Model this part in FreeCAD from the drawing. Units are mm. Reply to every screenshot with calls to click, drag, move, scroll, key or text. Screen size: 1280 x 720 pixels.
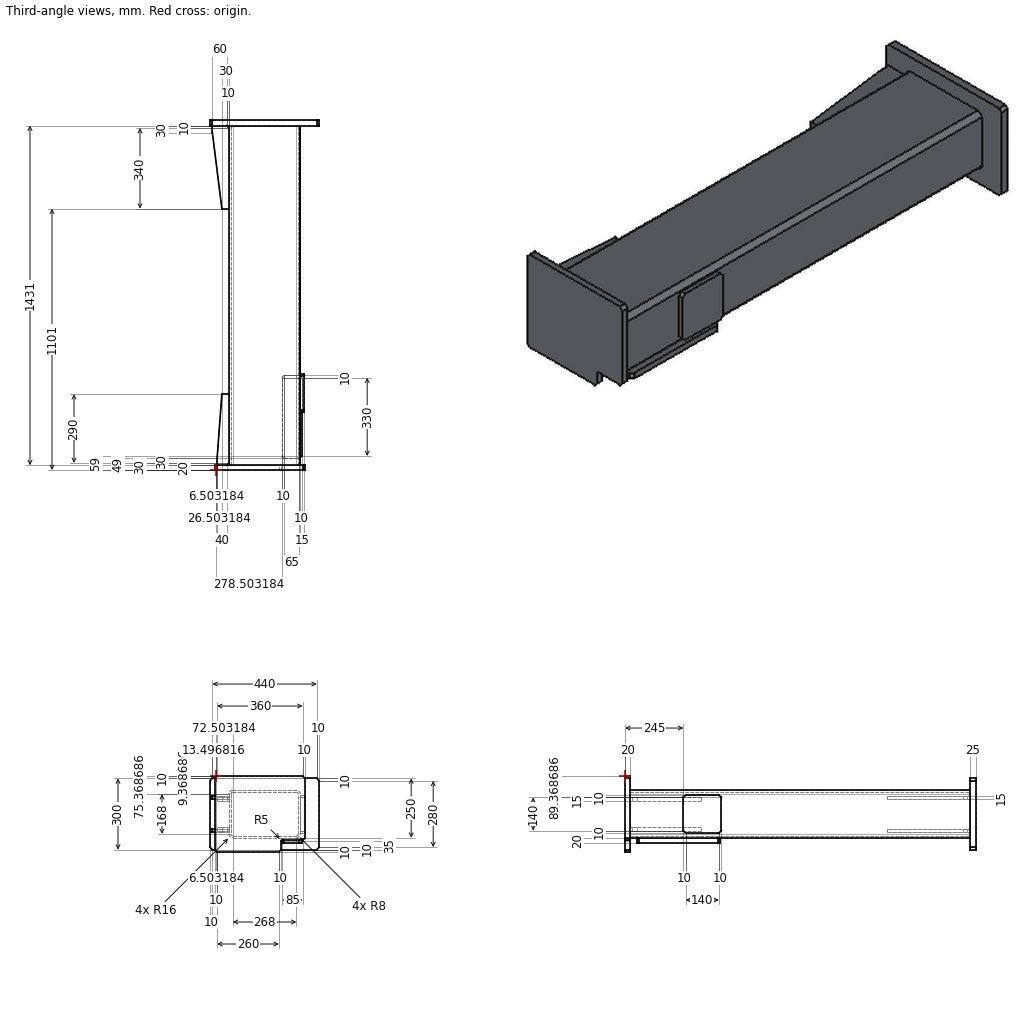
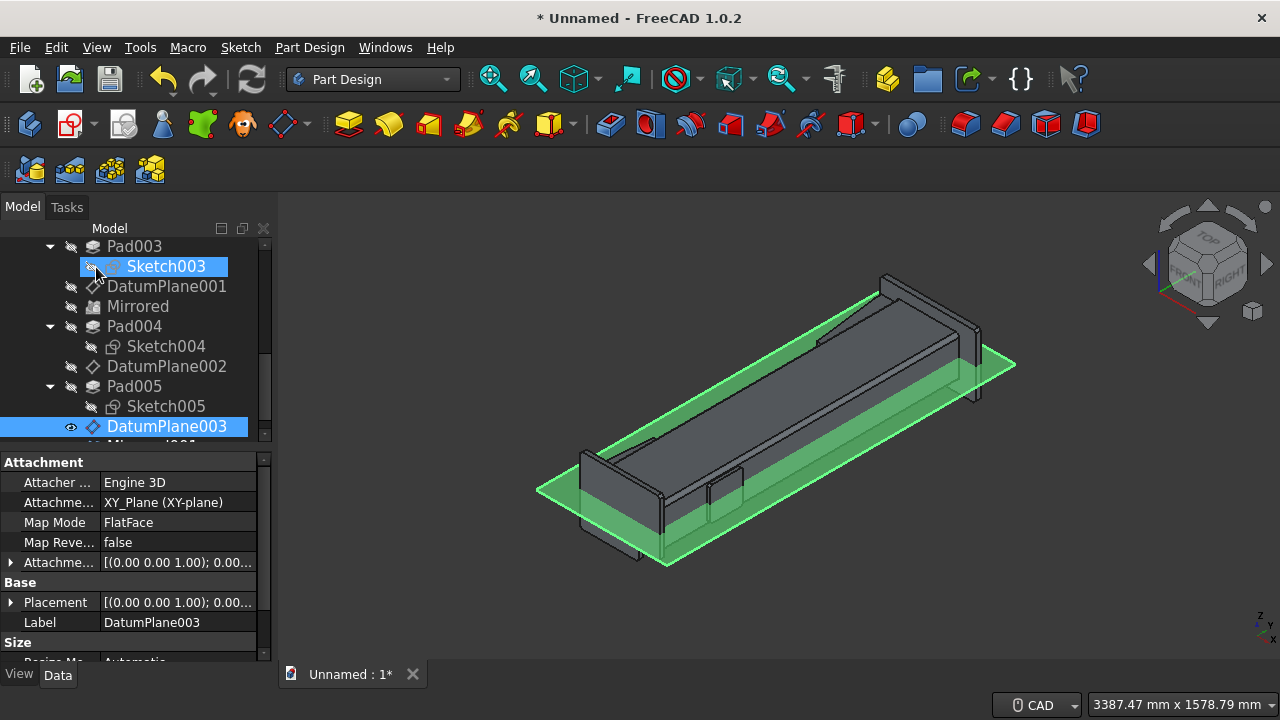
click(116, 427)
key(space)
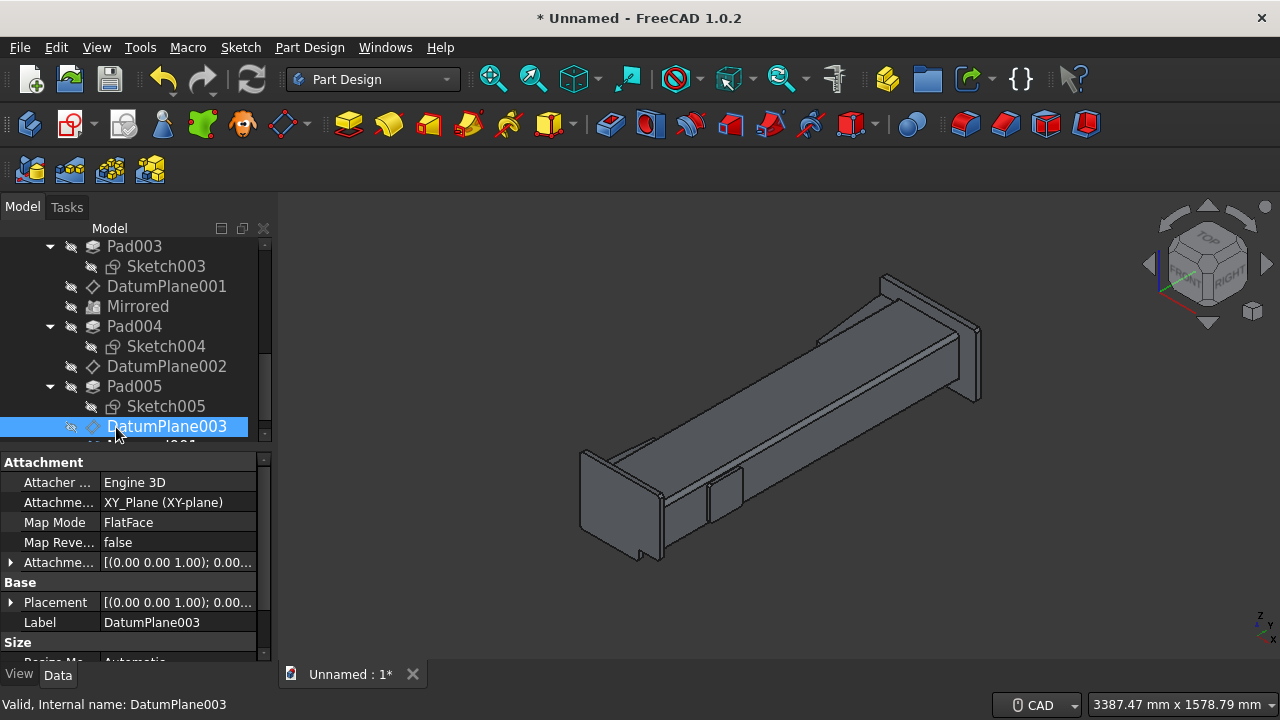
key(5)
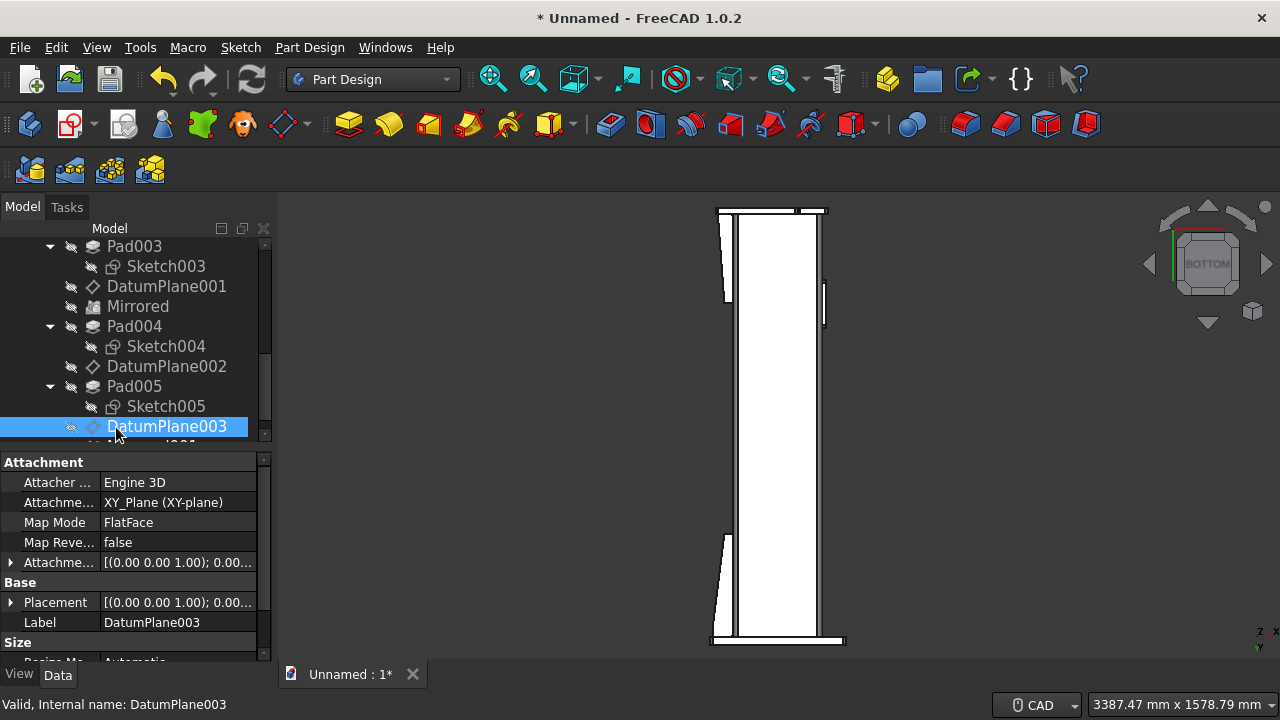
click(778, 545)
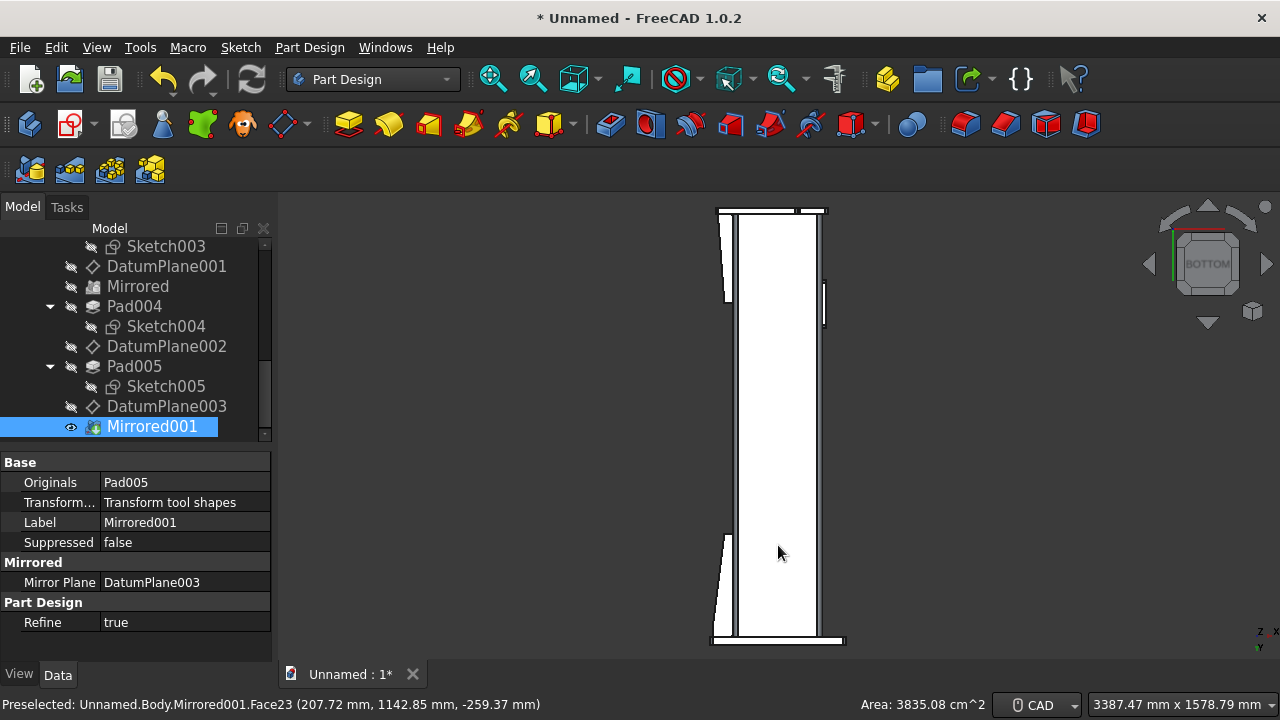
click(70, 124)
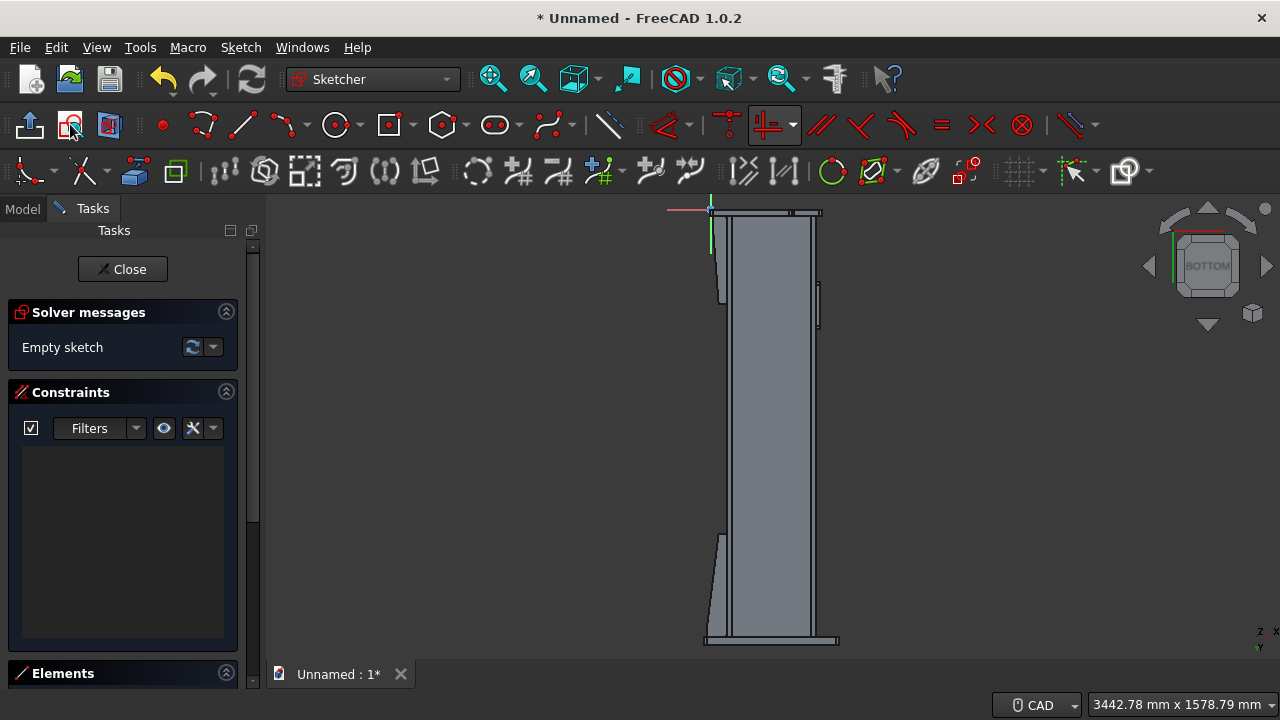
key(q)
key(s)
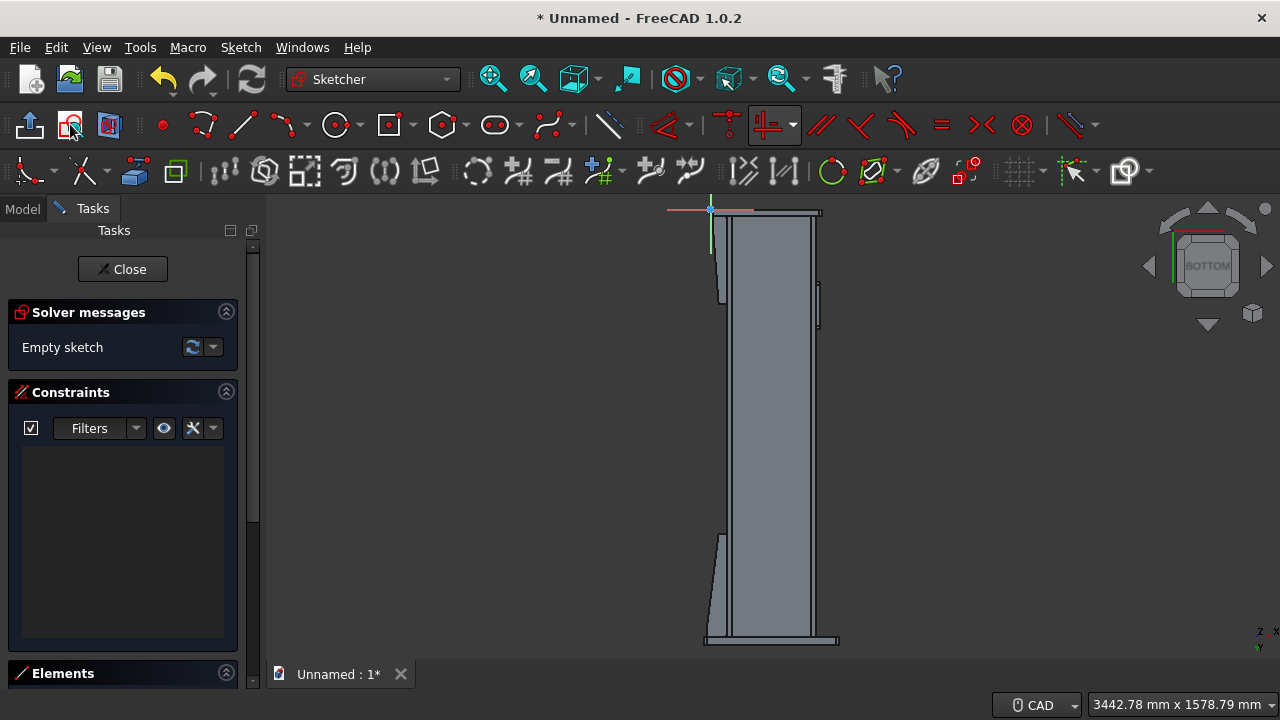
scroll(704, 426, down, 5)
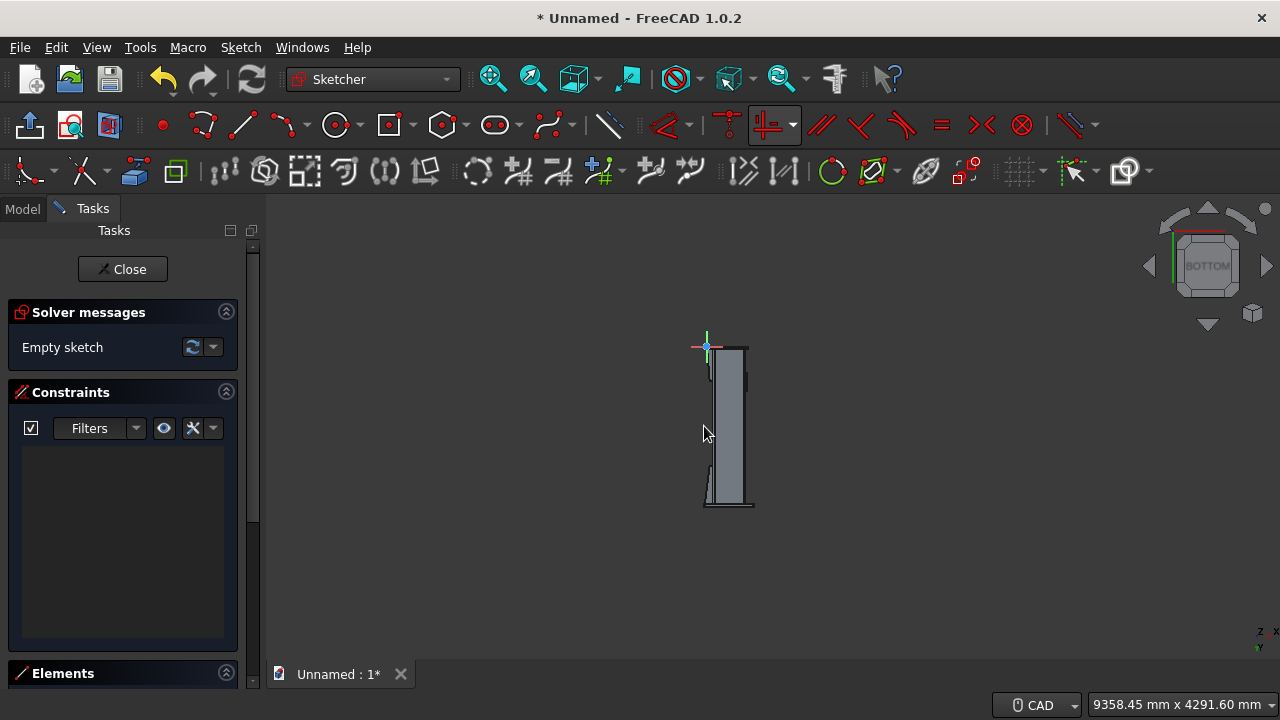
scroll(731, 357, up, 9)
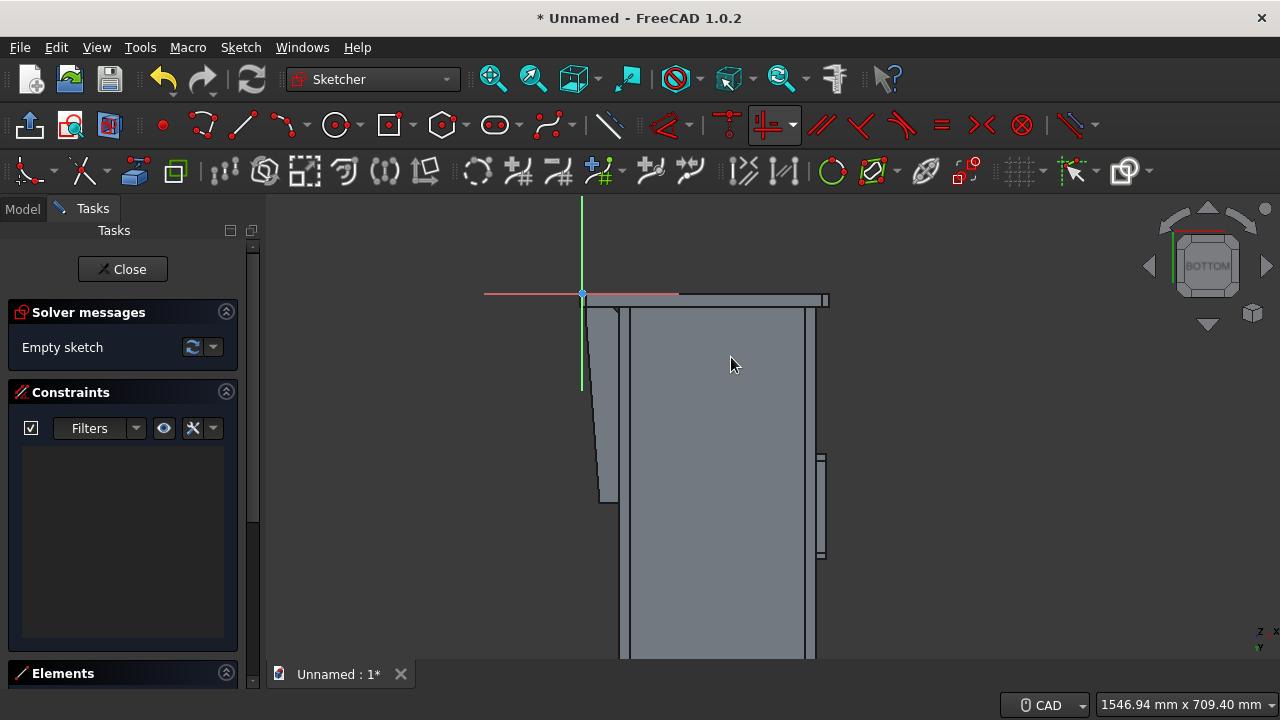
click(204, 126)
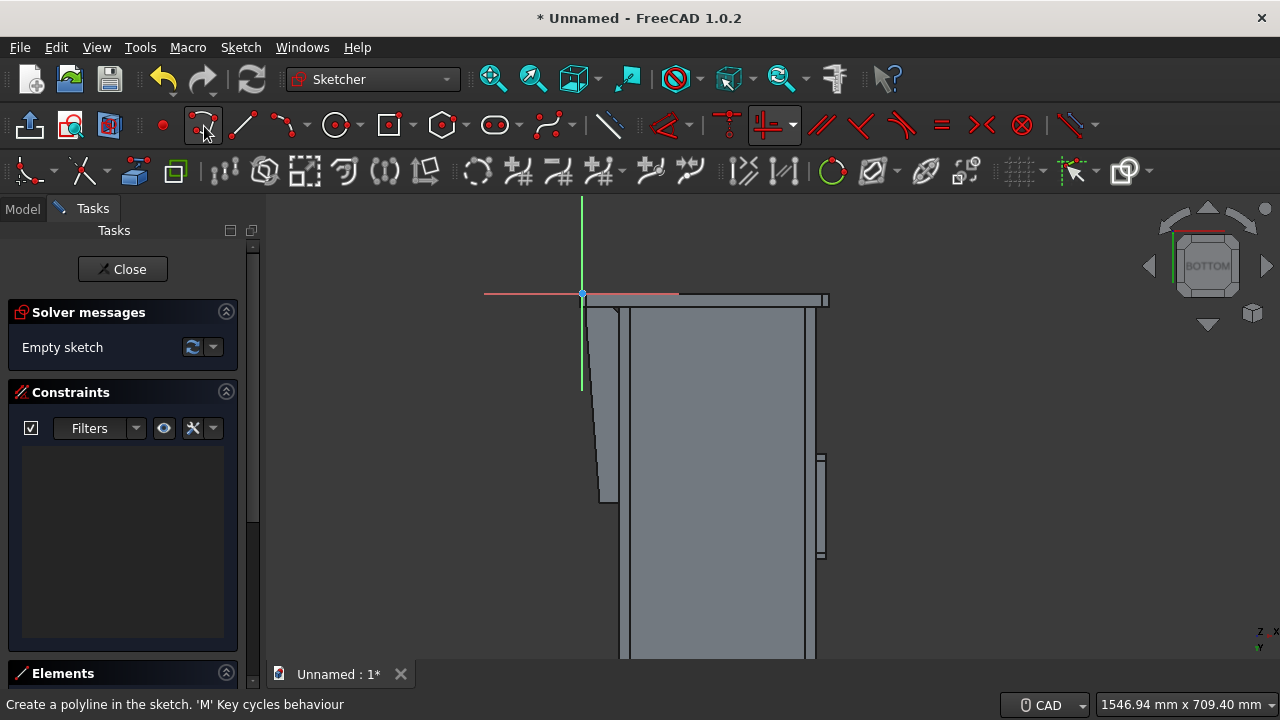
click(765, 332)
click(765, 549)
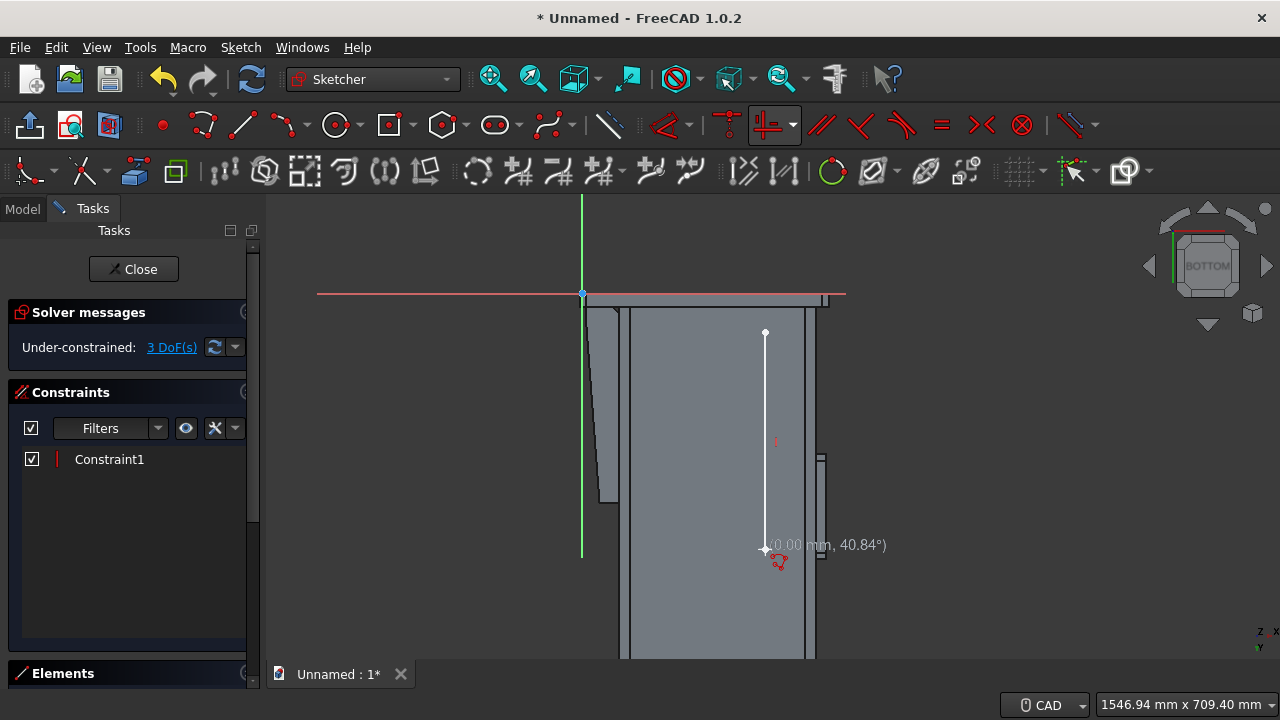
scroll(771, 555, up, 3)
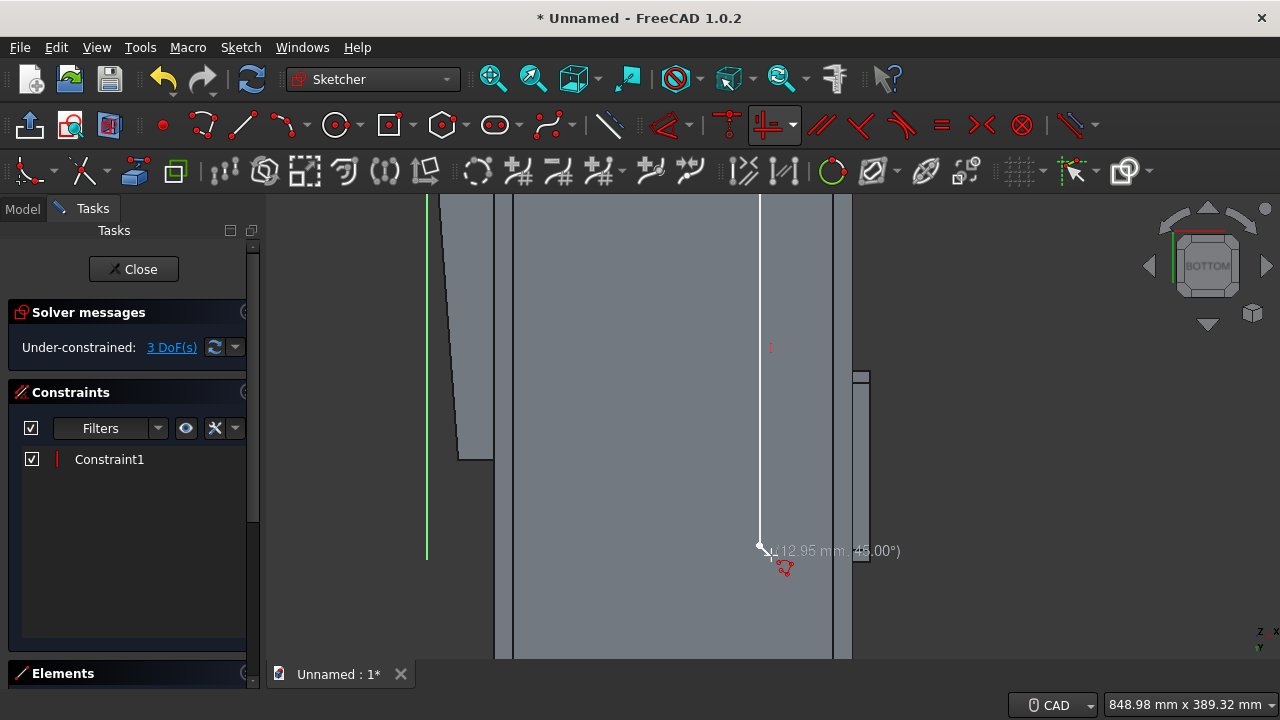
click(771, 555)
click(849, 555)
click(861, 543)